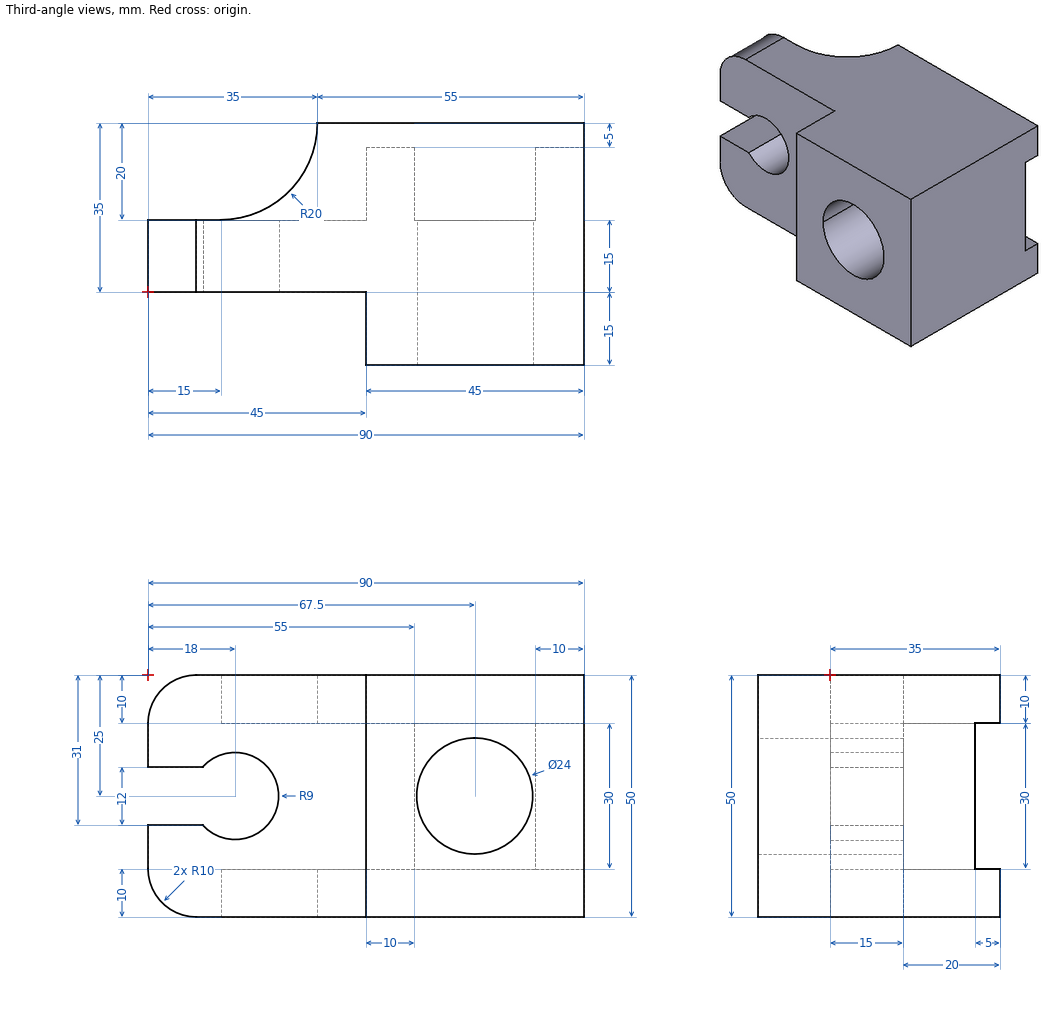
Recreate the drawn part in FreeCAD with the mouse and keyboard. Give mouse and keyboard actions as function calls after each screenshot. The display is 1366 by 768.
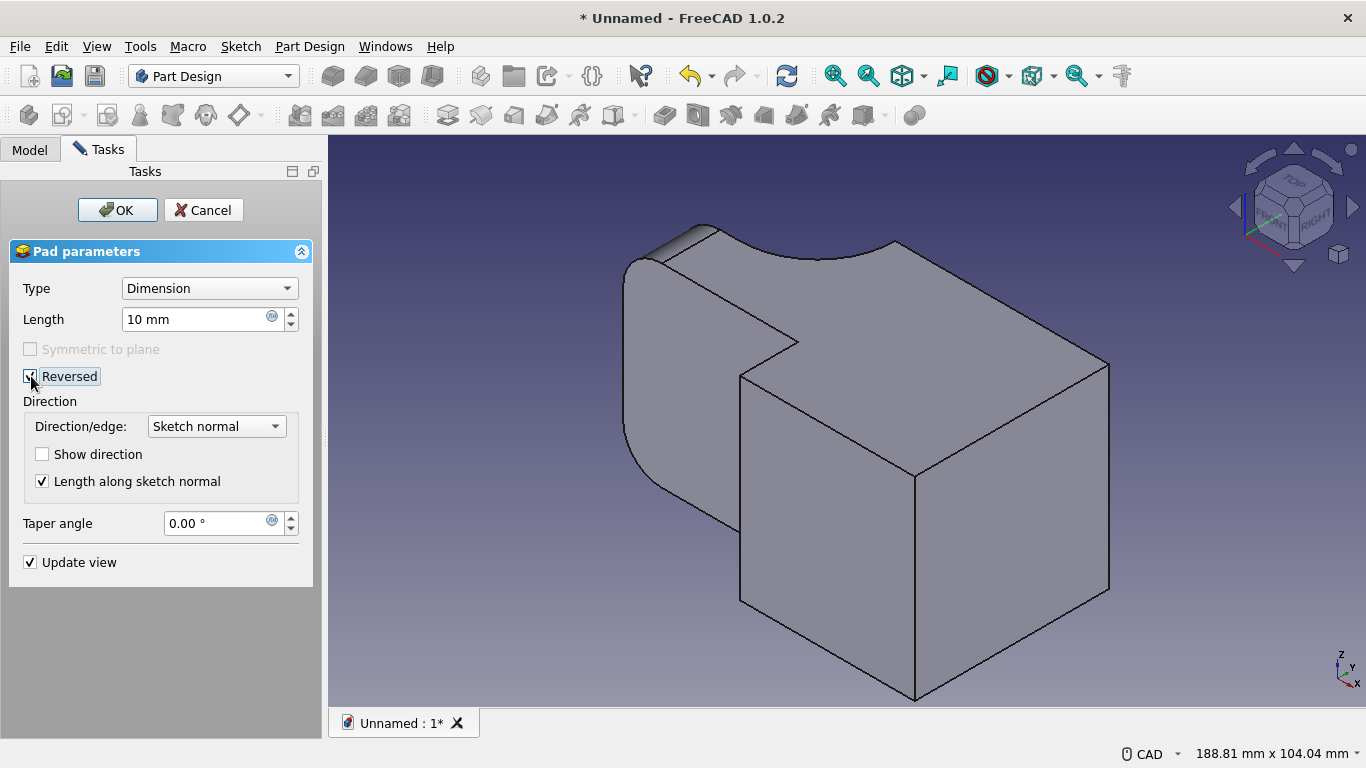
click(118, 210)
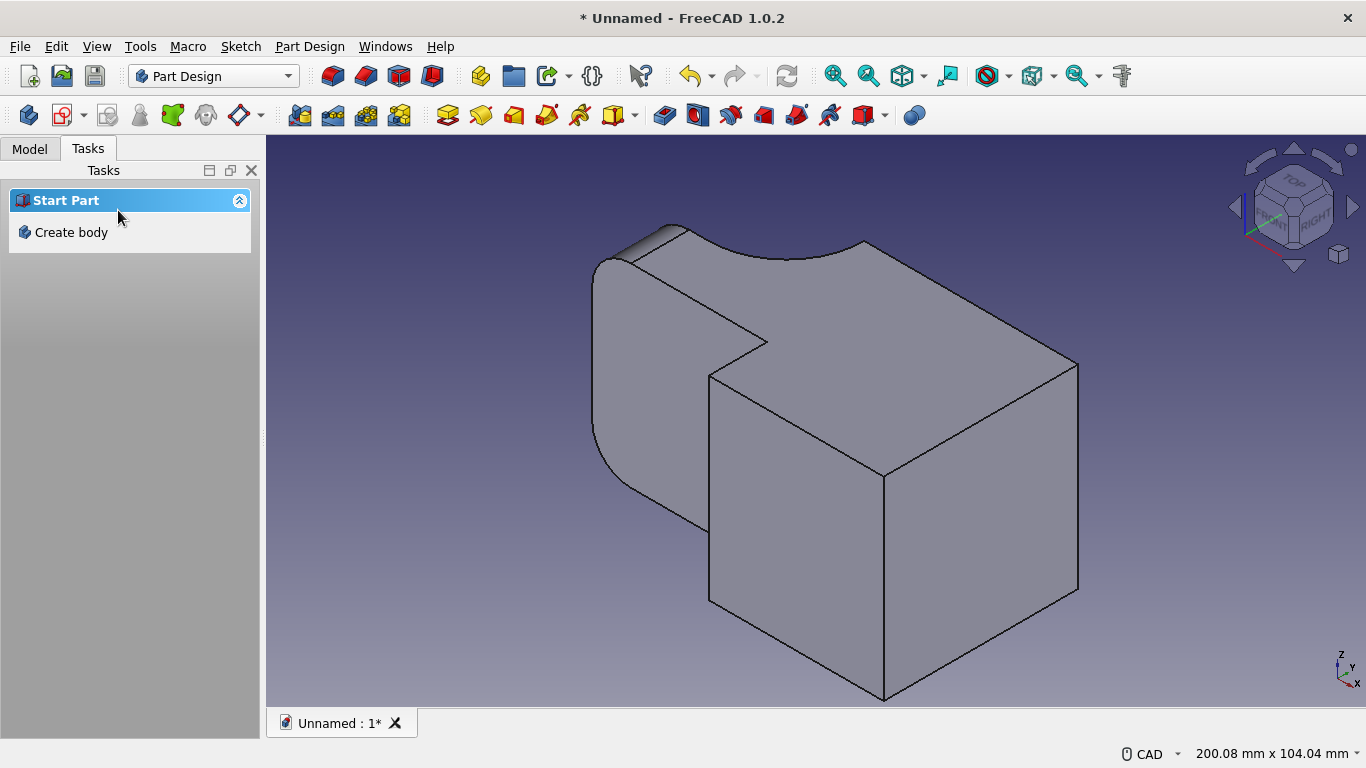
click(30, 148)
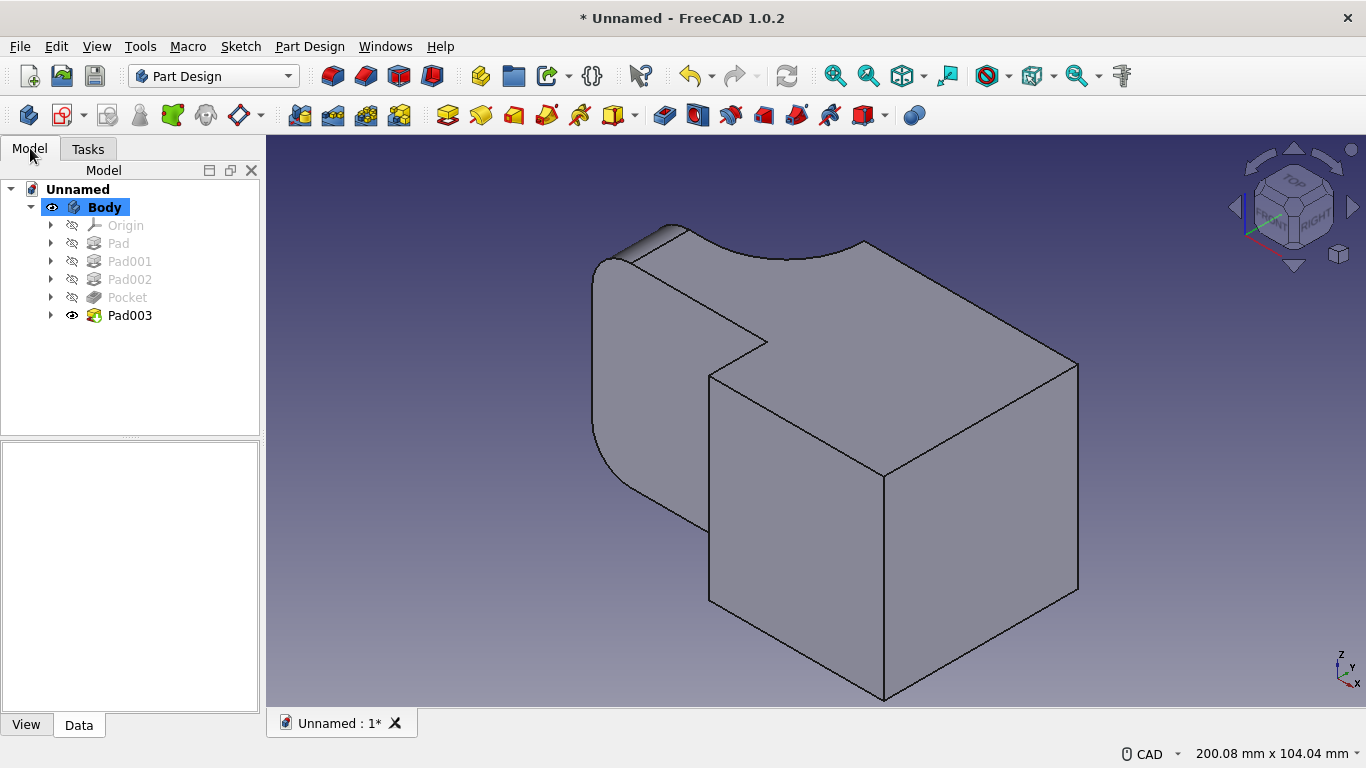
click(51, 225)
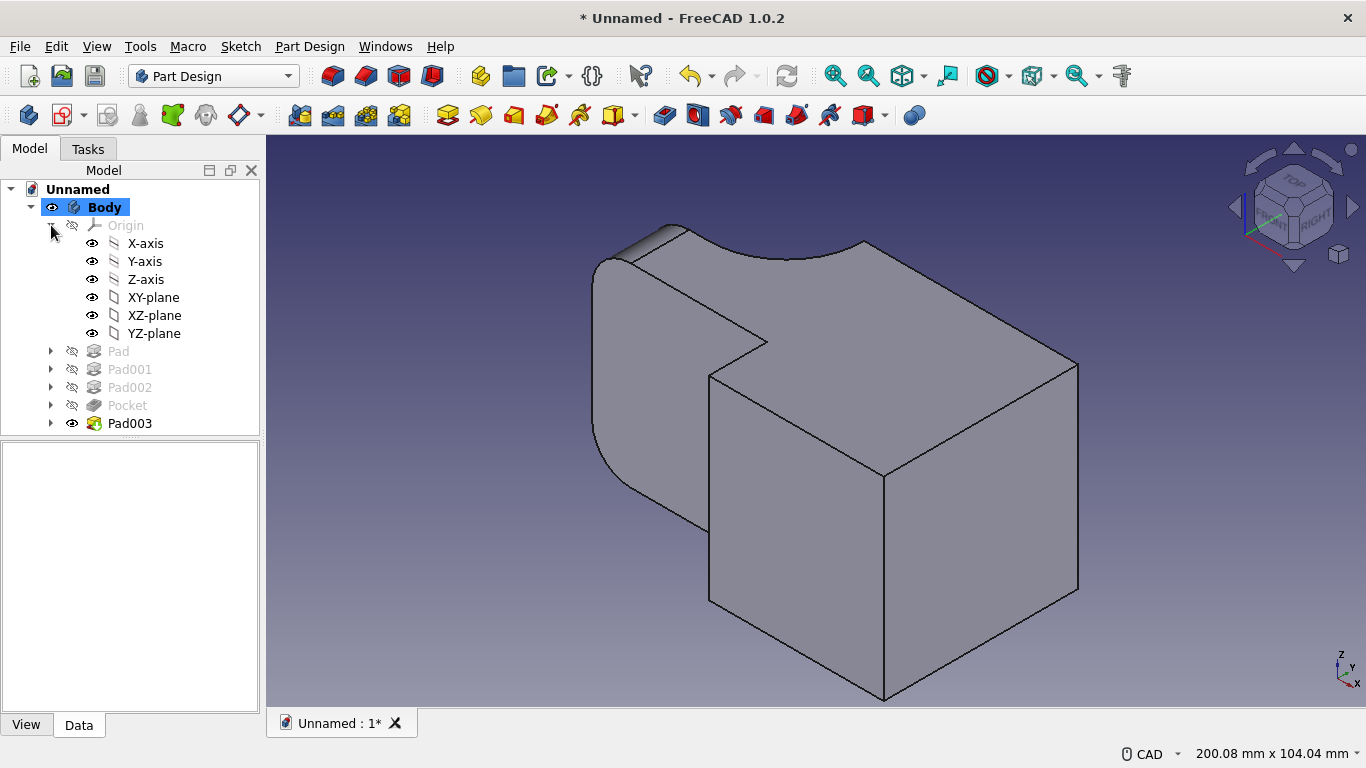
click(137, 297)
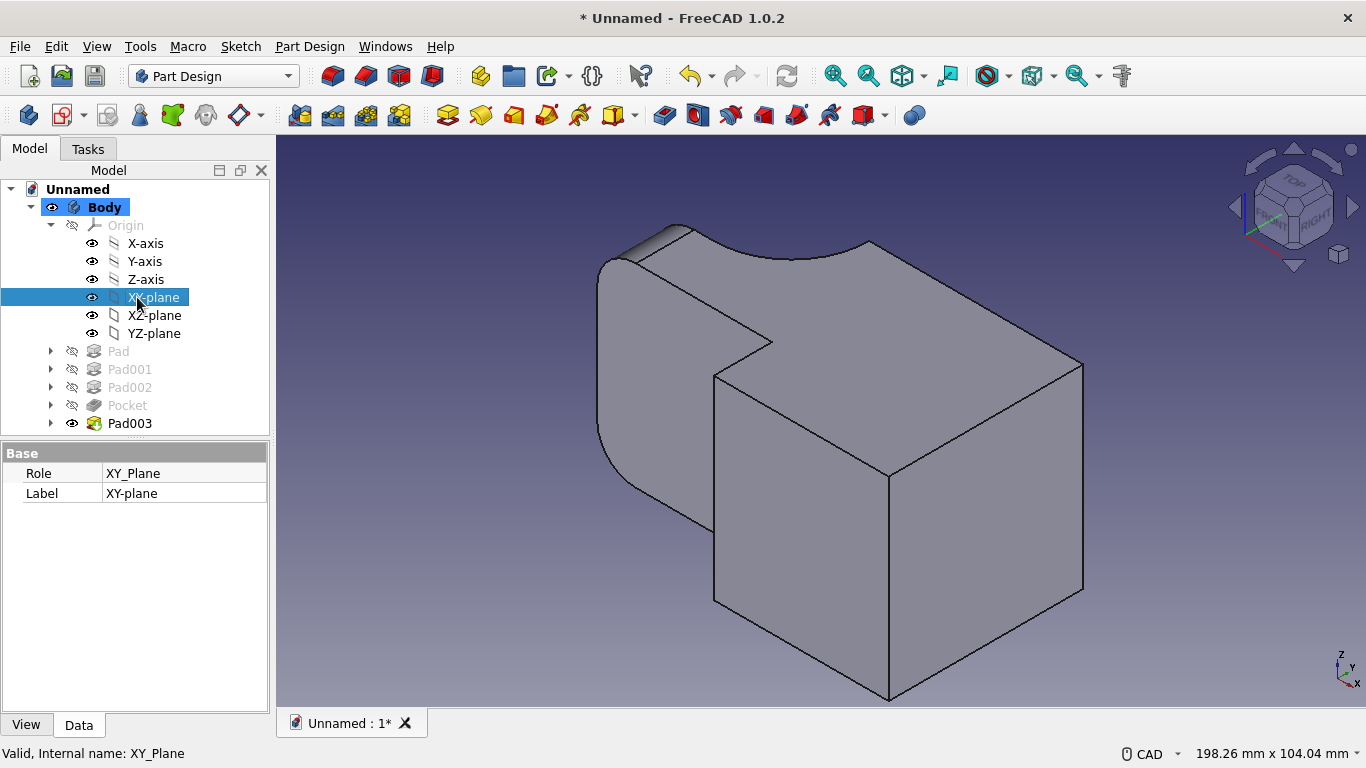
click(238, 116)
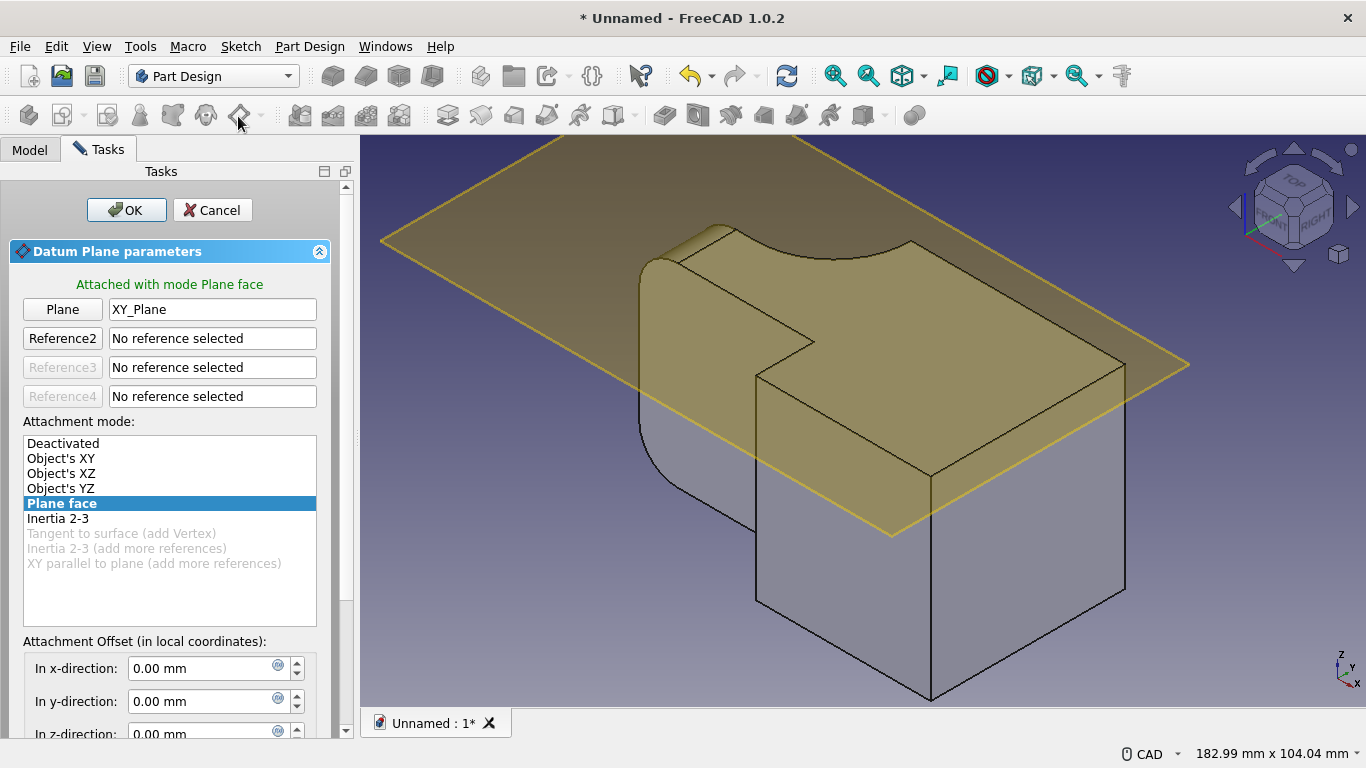
scroll(346, 460, down, 2)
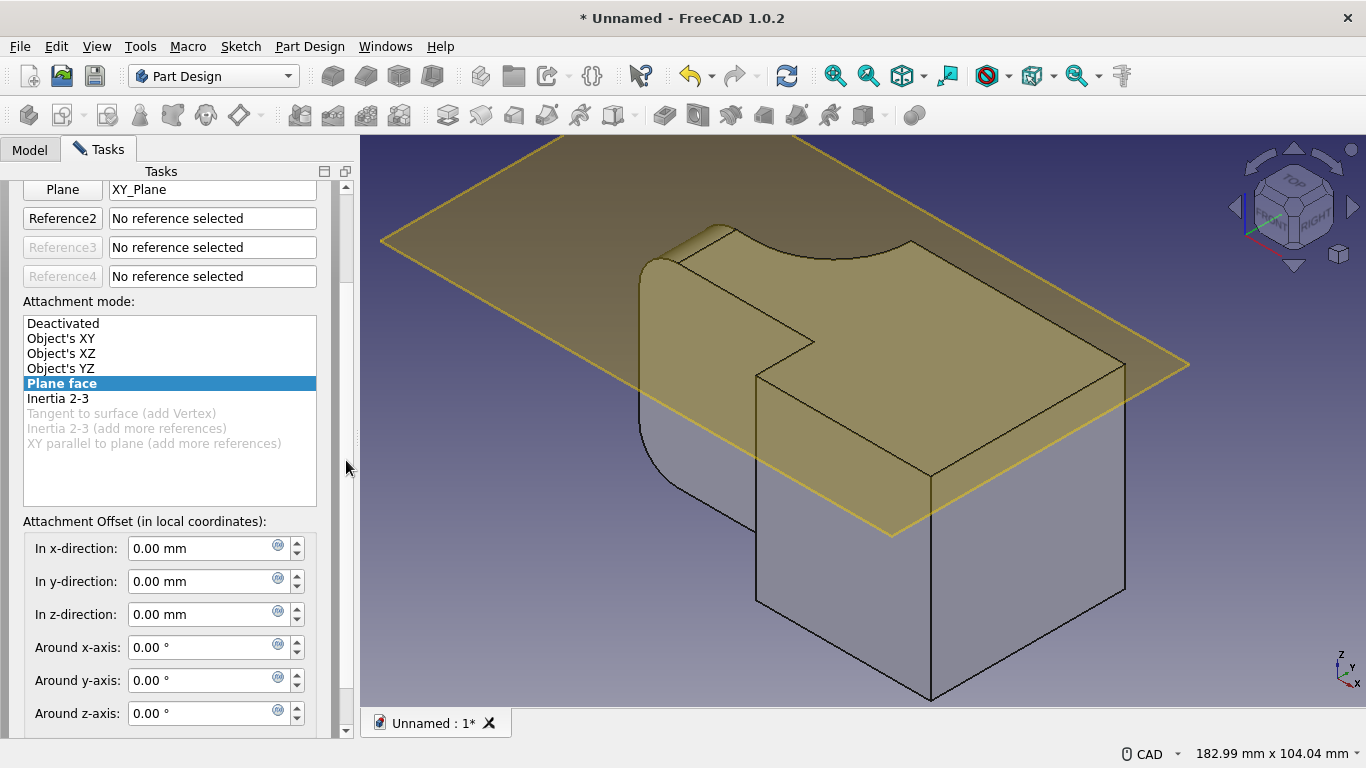
triple_click(210, 614)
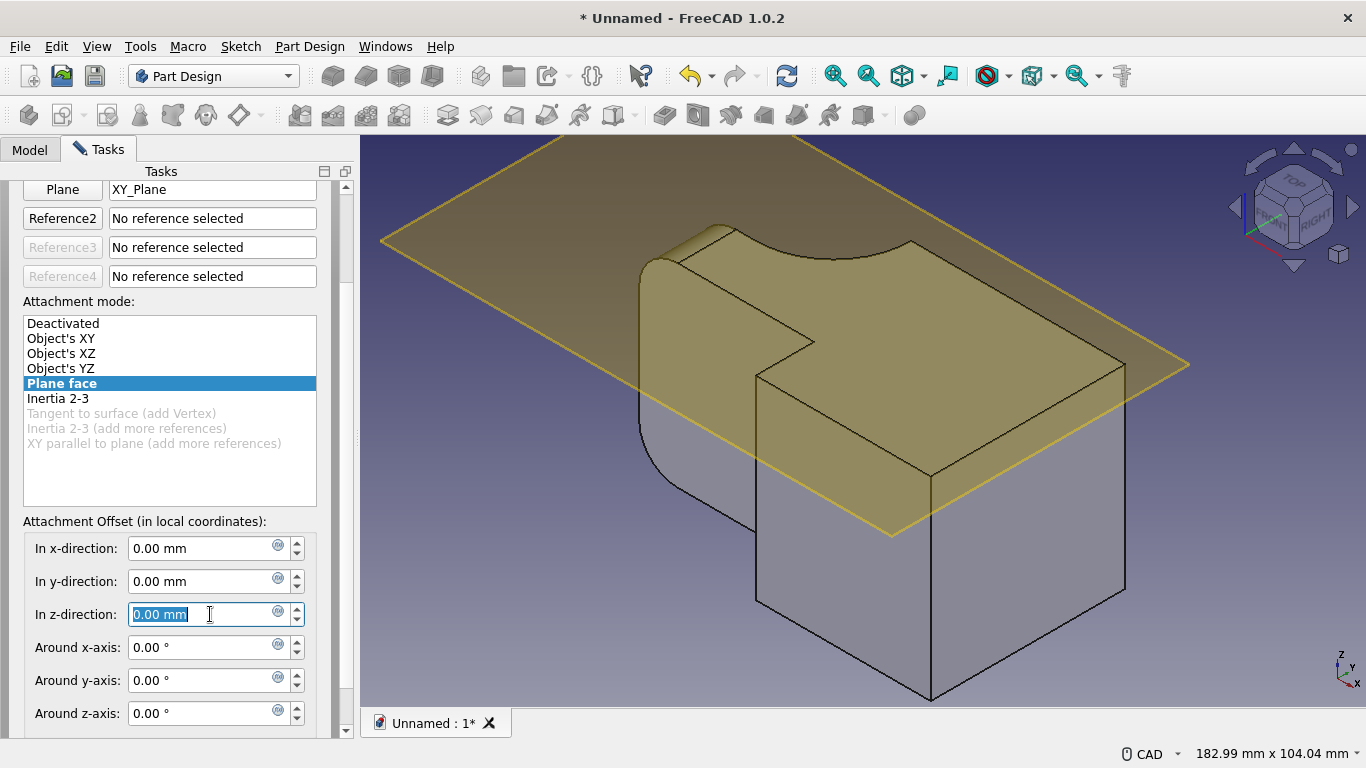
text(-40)
key(Tab)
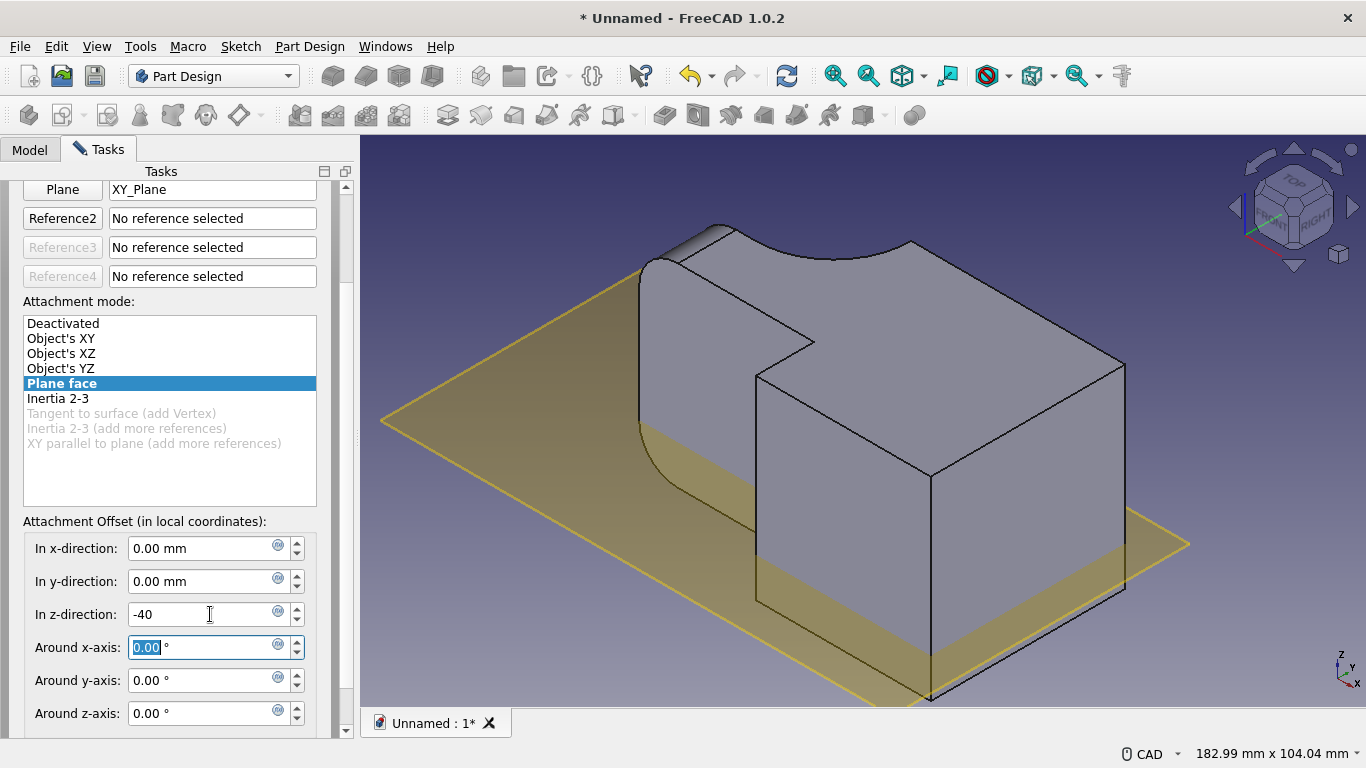
scroll(346, 460, up, 3)